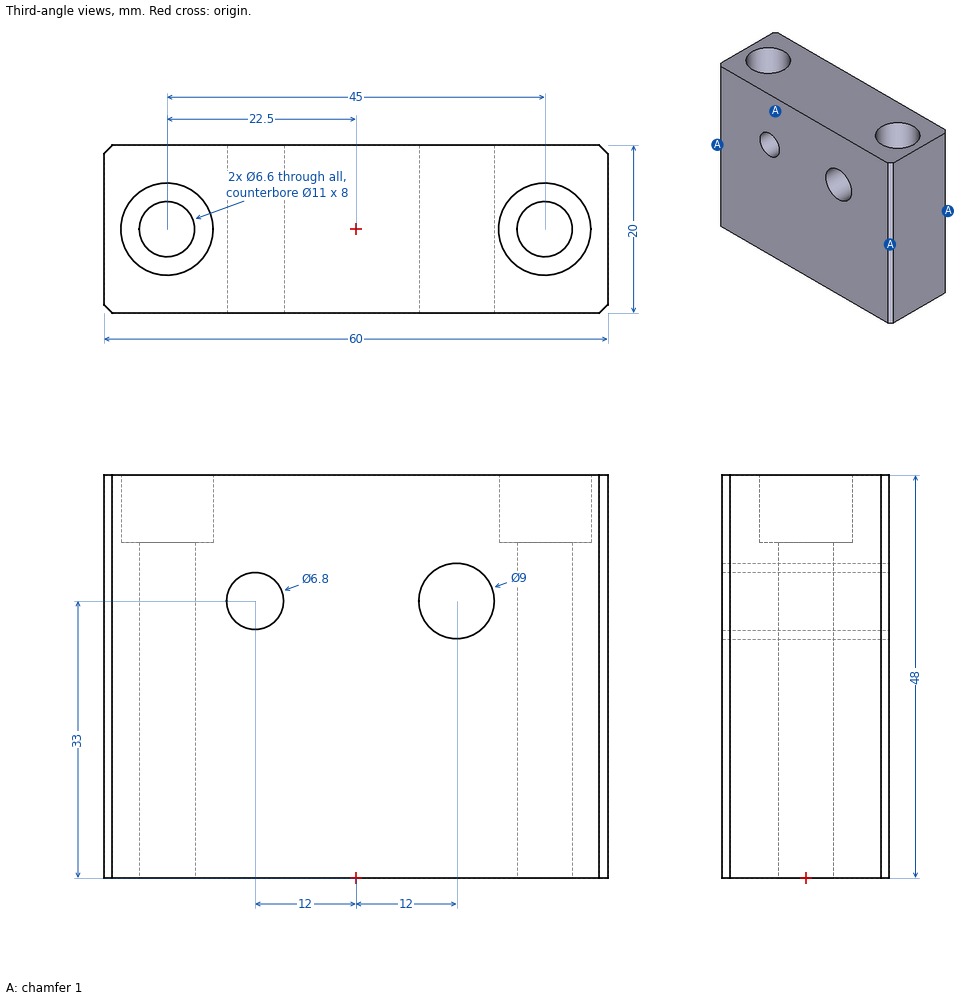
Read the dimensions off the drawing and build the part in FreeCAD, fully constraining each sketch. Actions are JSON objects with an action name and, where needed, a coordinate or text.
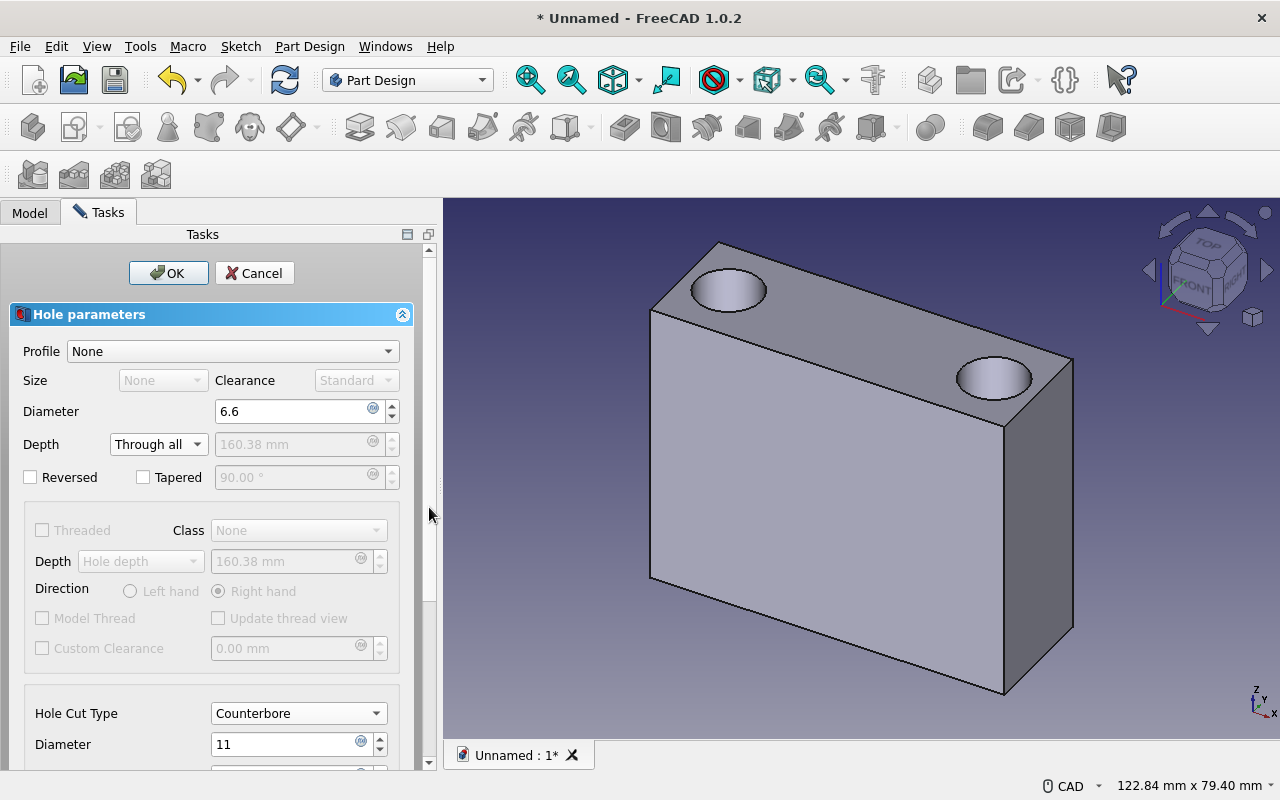
{"action": "left_click", "coordinate": [169, 273]}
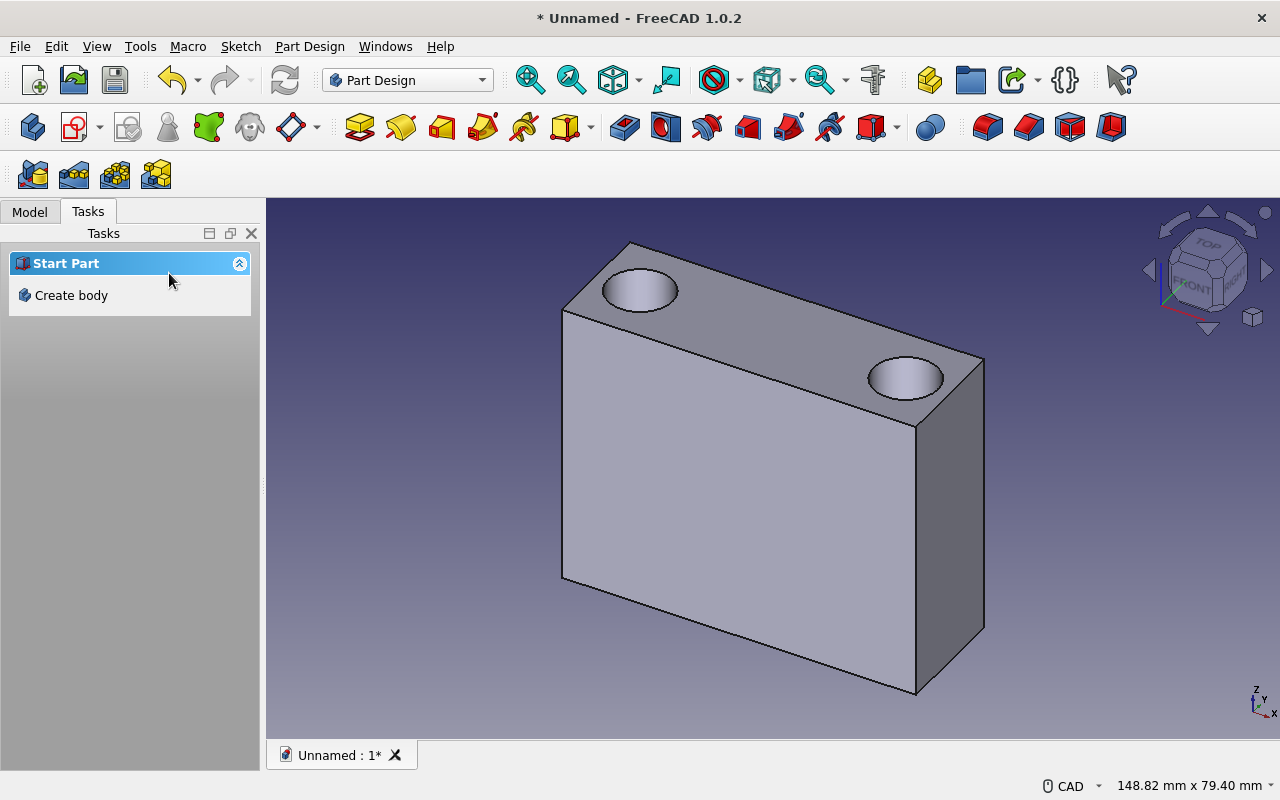
{"action": "left_click", "coordinate": [739, 501]}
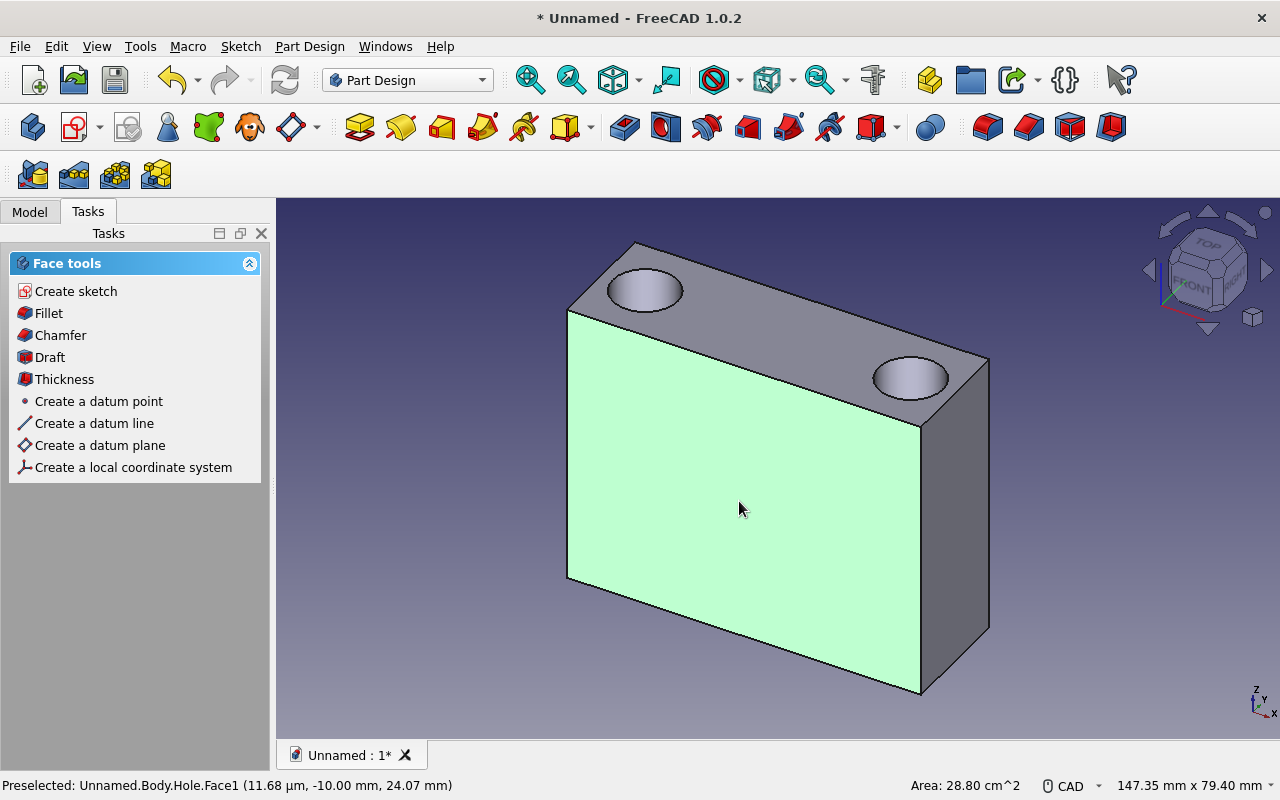
{"action": "left_click", "coordinate": [74, 128]}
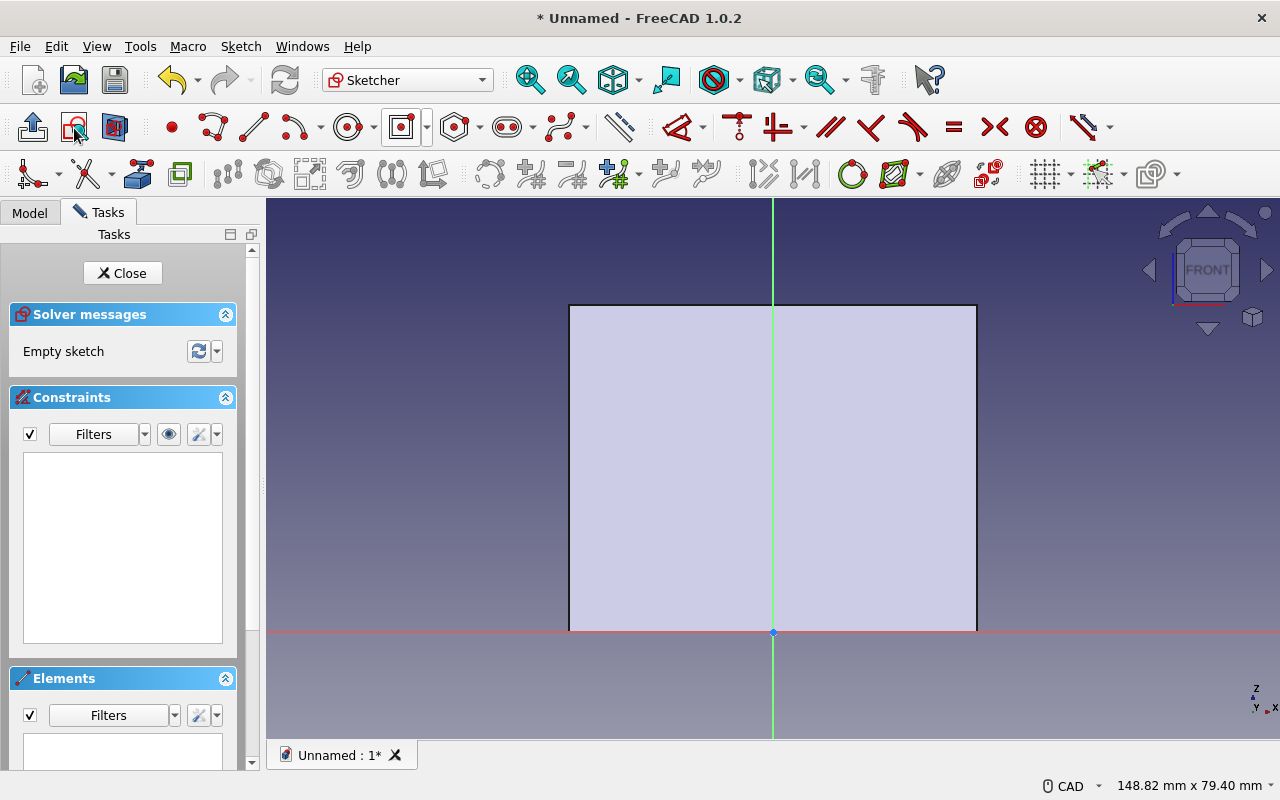
{"action": "scroll", "coordinate": [689, 398], "scroll_direction": "up", "scroll_amount": 10}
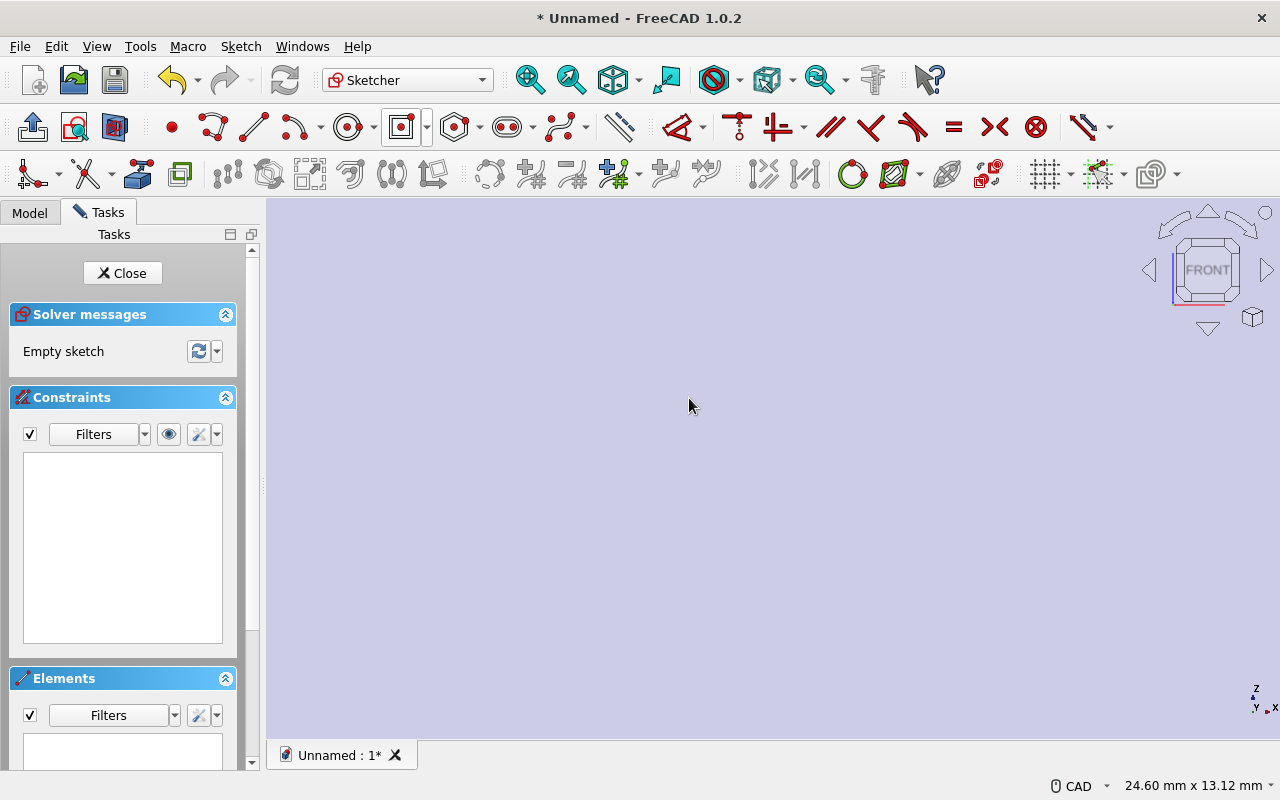
{"action": "left_click", "coordinate": [348, 128]}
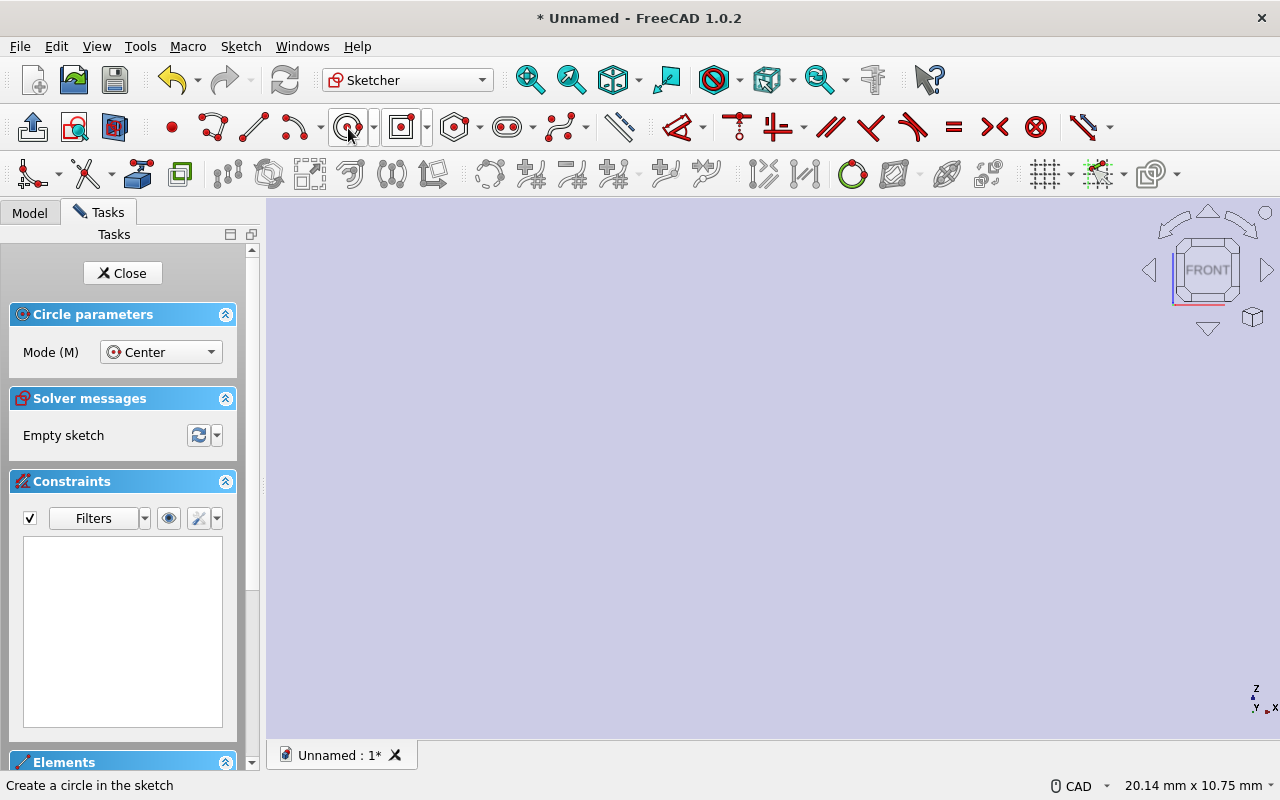
{"action": "left_click", "coordinate": [703, 463]}
{"action": "mouse_move", "coordinate": [824, 342]}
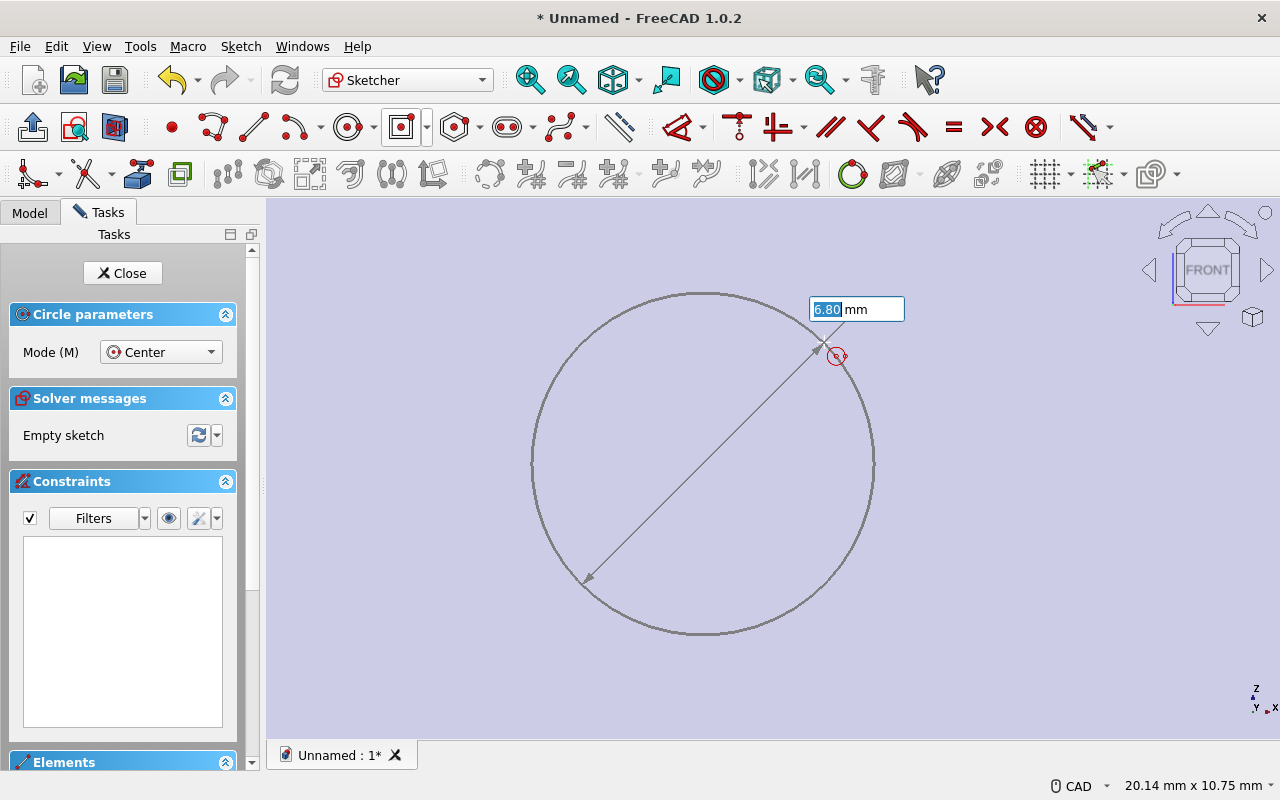
{"action": "type", "text": "6.8"}
{"action": "key", "text": "Return"}
{"action": "key", "text": "Escape"}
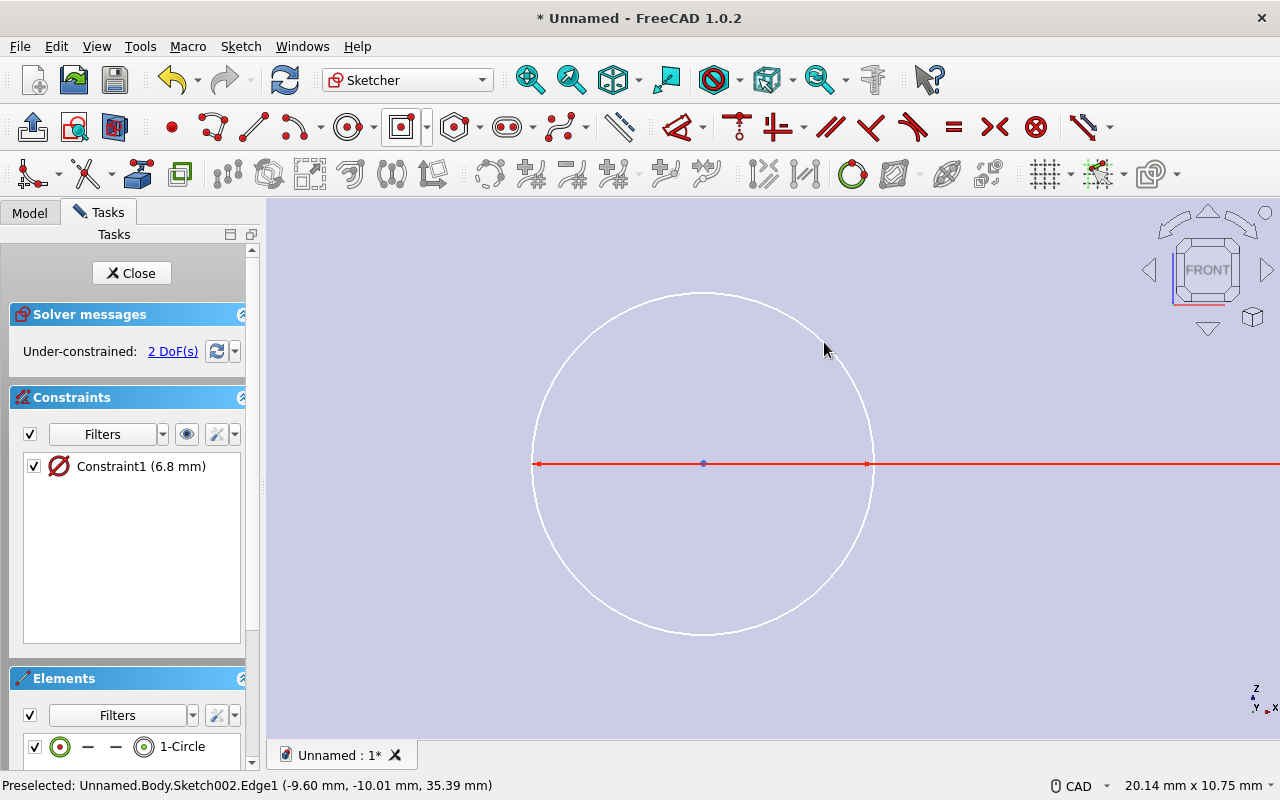
{"action": "left_click", "coordinate": [676, 128]}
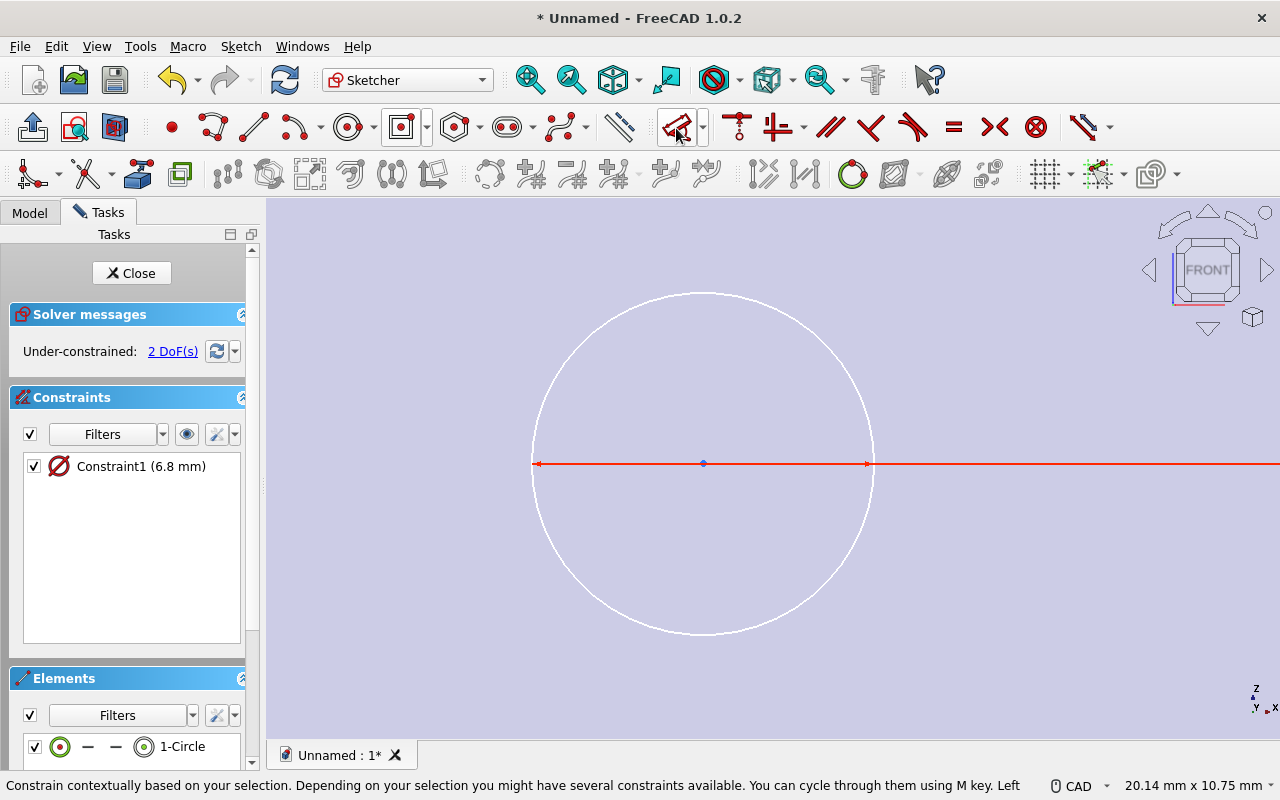
{"action": "left_click", "coordinate": [703, 464]}
{"action": "left_click", "coordinate": [909, 430]}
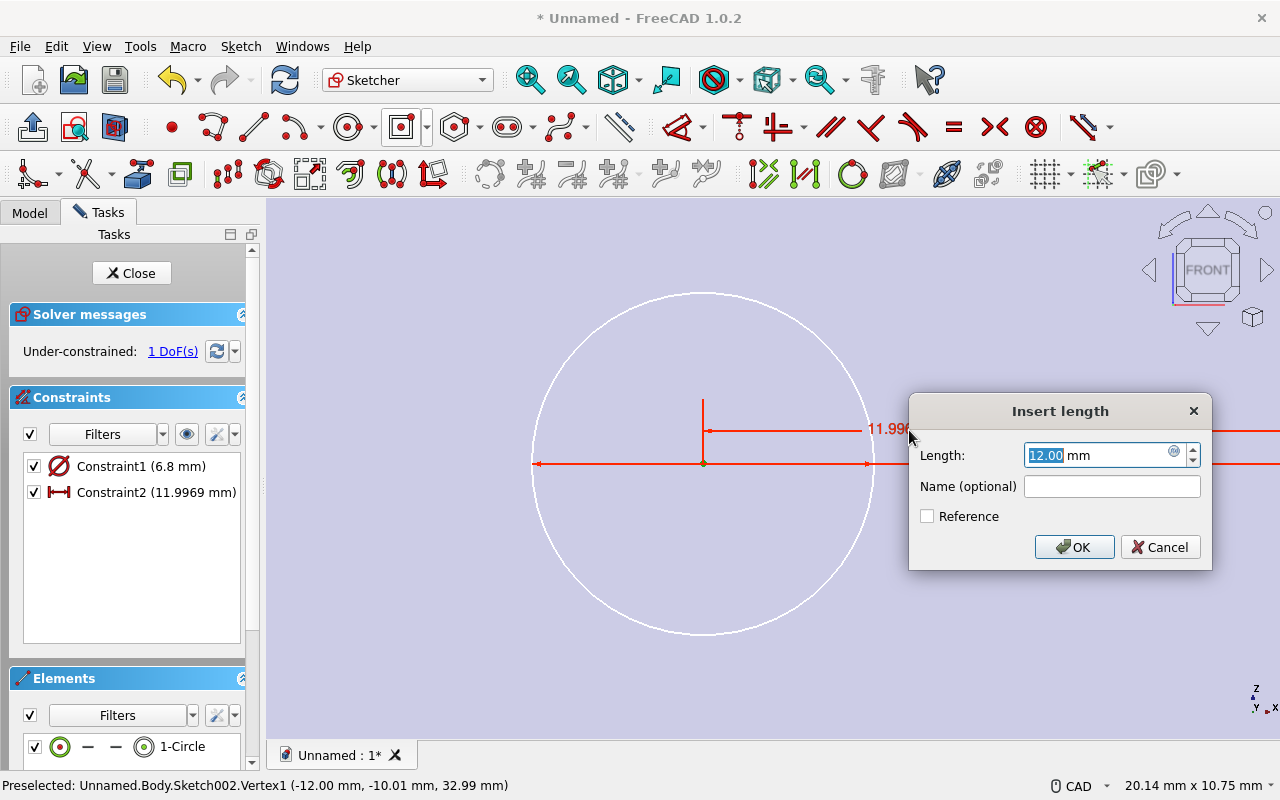
{"action": "type", "text": "12"}
{"action": "key", "text": "Return"}